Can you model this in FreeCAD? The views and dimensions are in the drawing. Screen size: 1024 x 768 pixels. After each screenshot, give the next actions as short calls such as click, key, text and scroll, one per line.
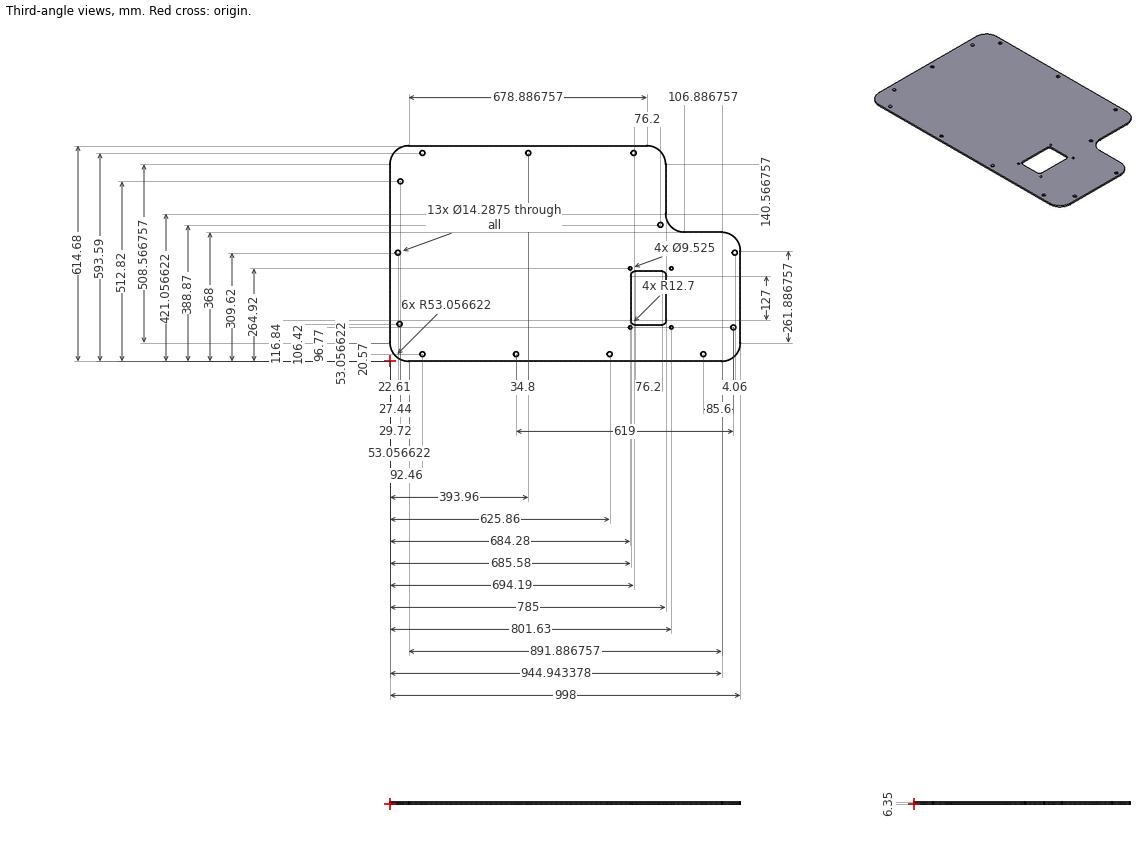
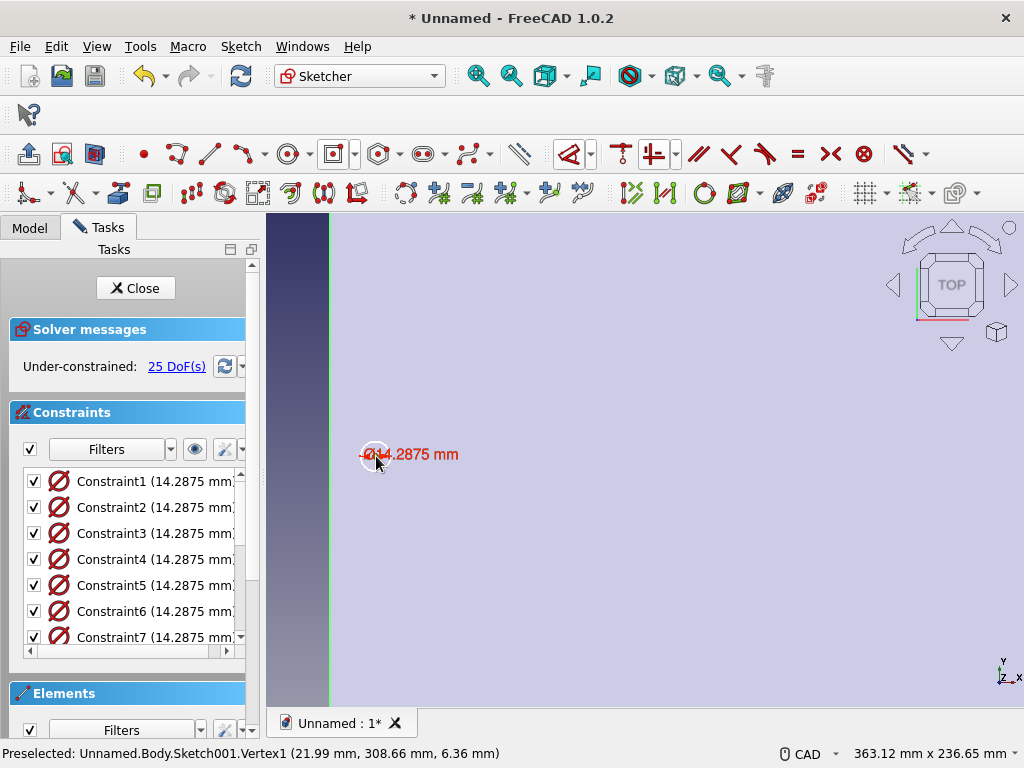
key(l)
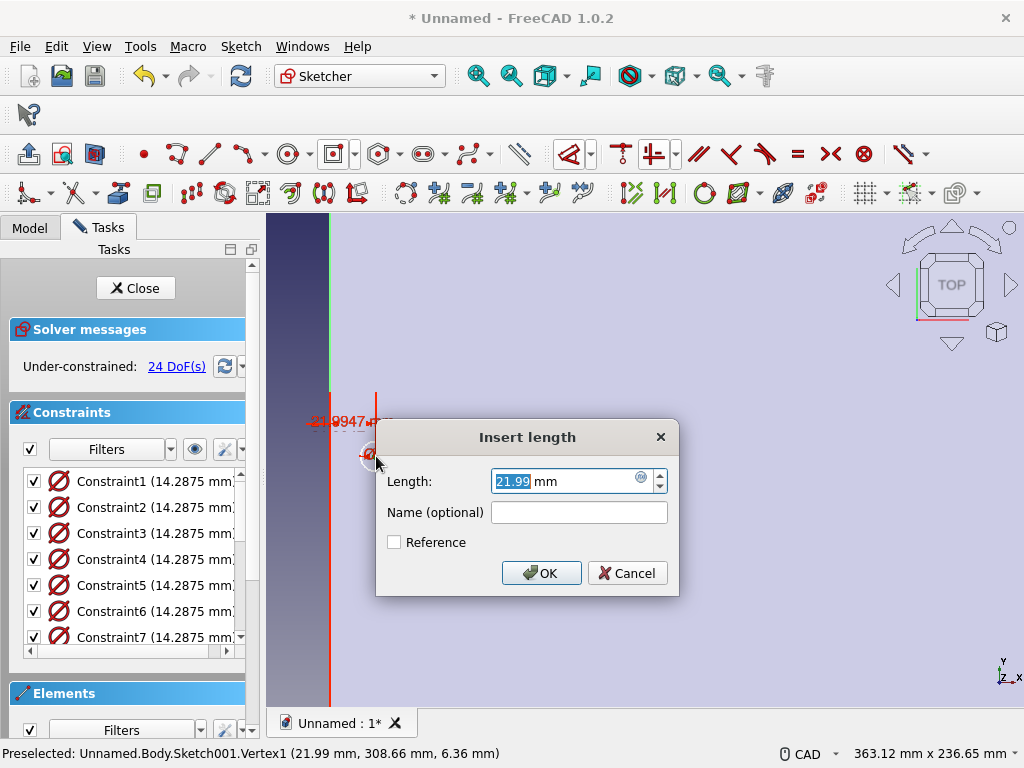
text(22.61)
key(Return)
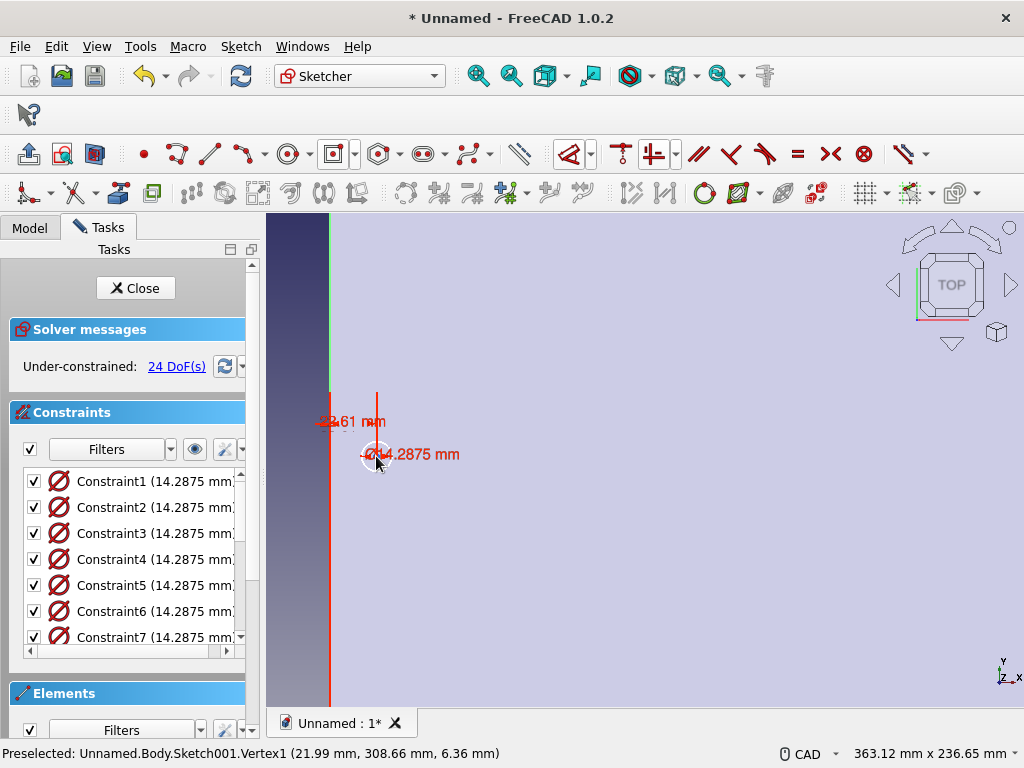
scroll(378, 457, down, 8)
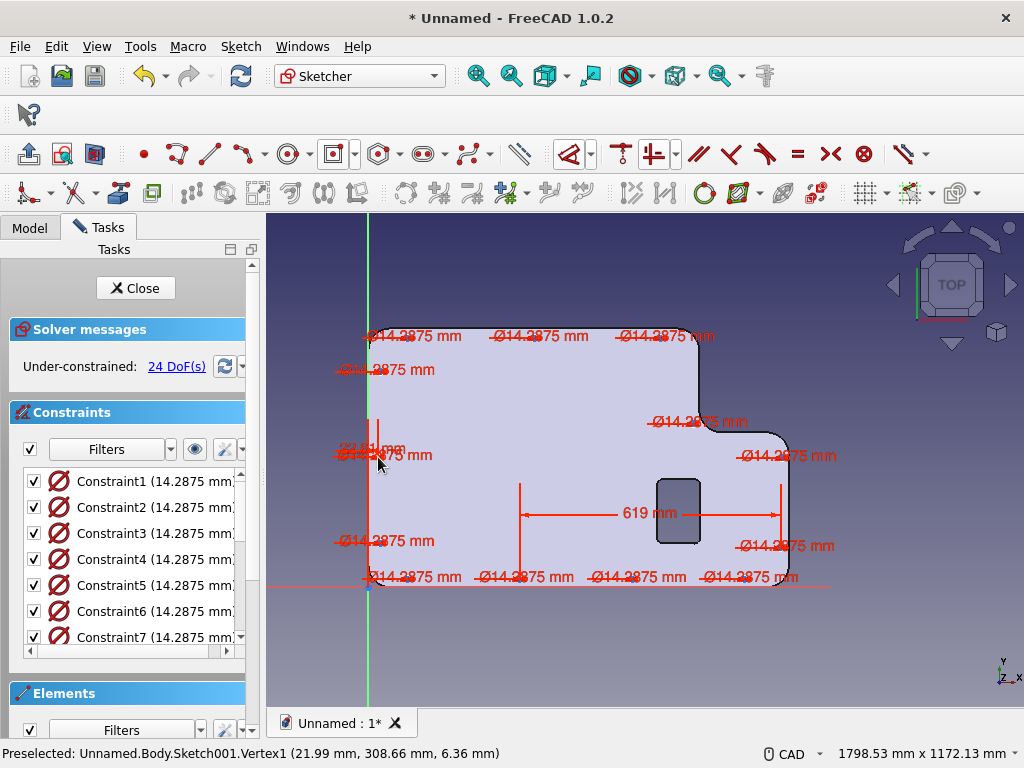
scroll(381, 372, up, 6)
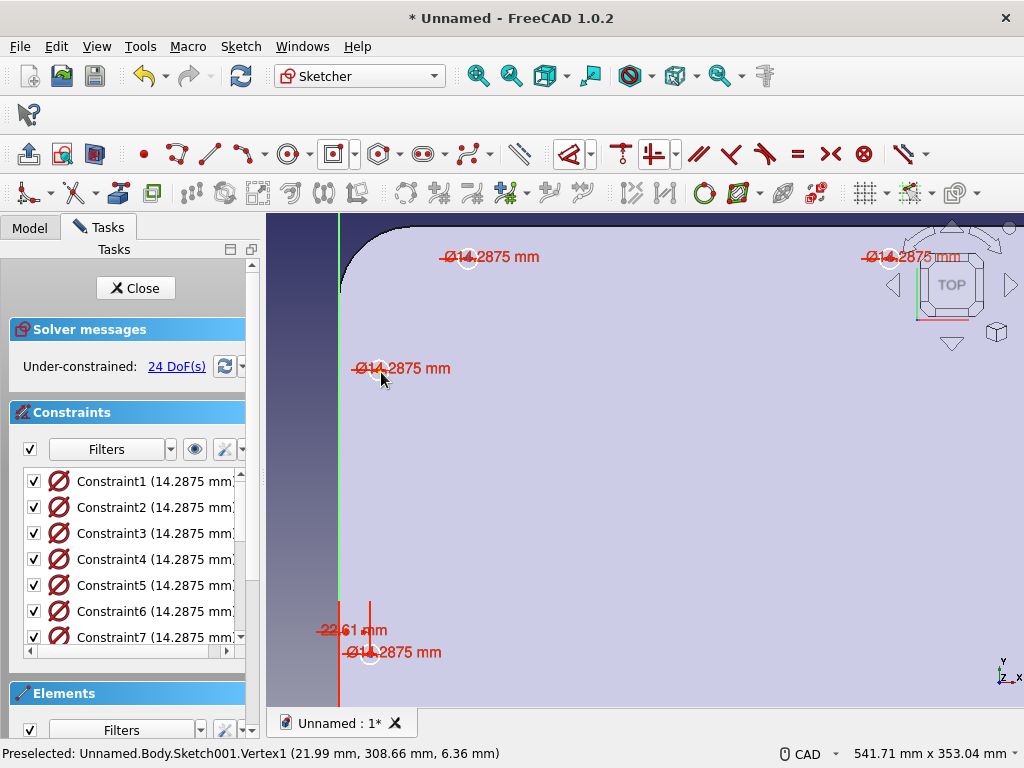
click(379, 370)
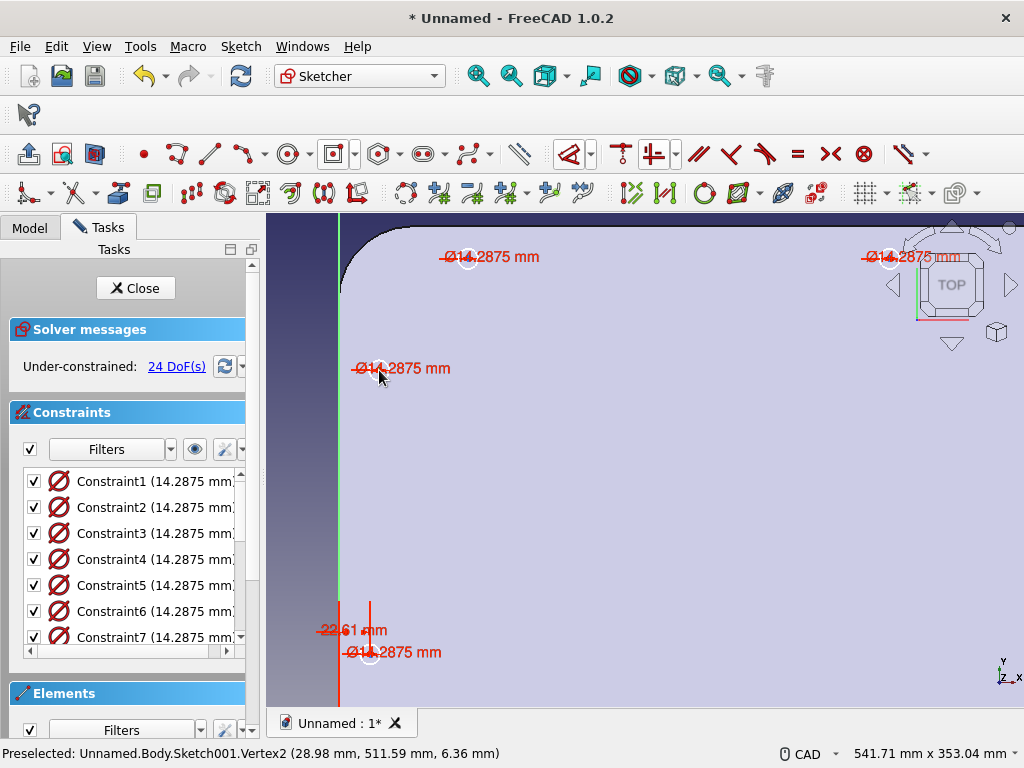
click(590, 154)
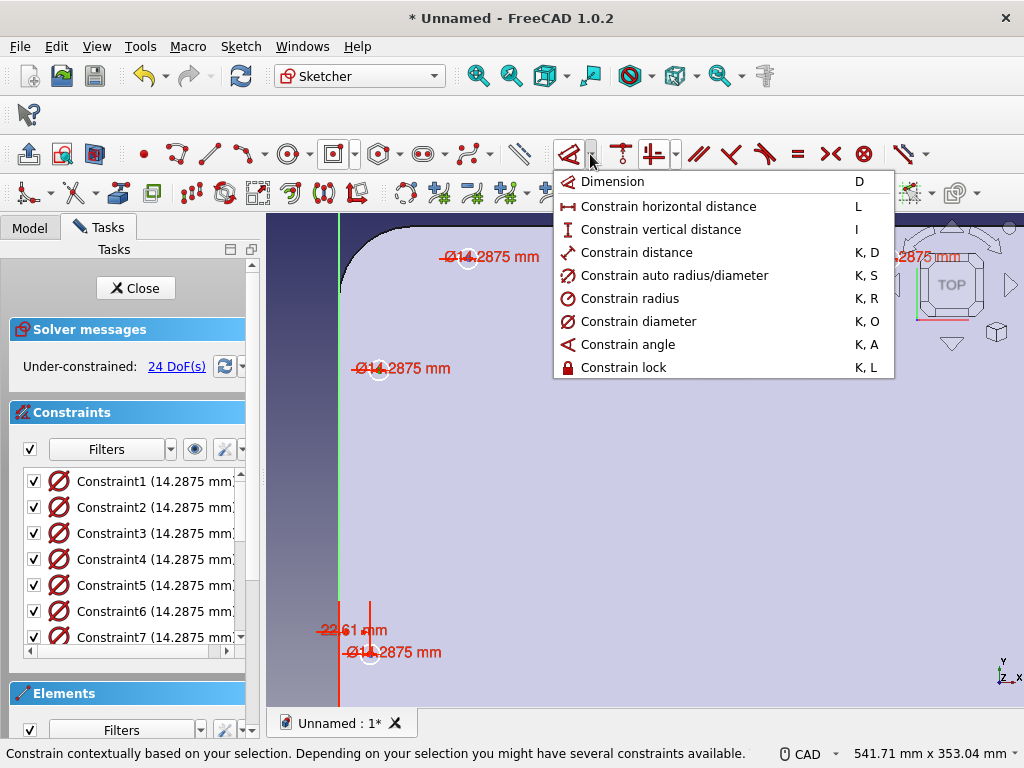
click(724, 206)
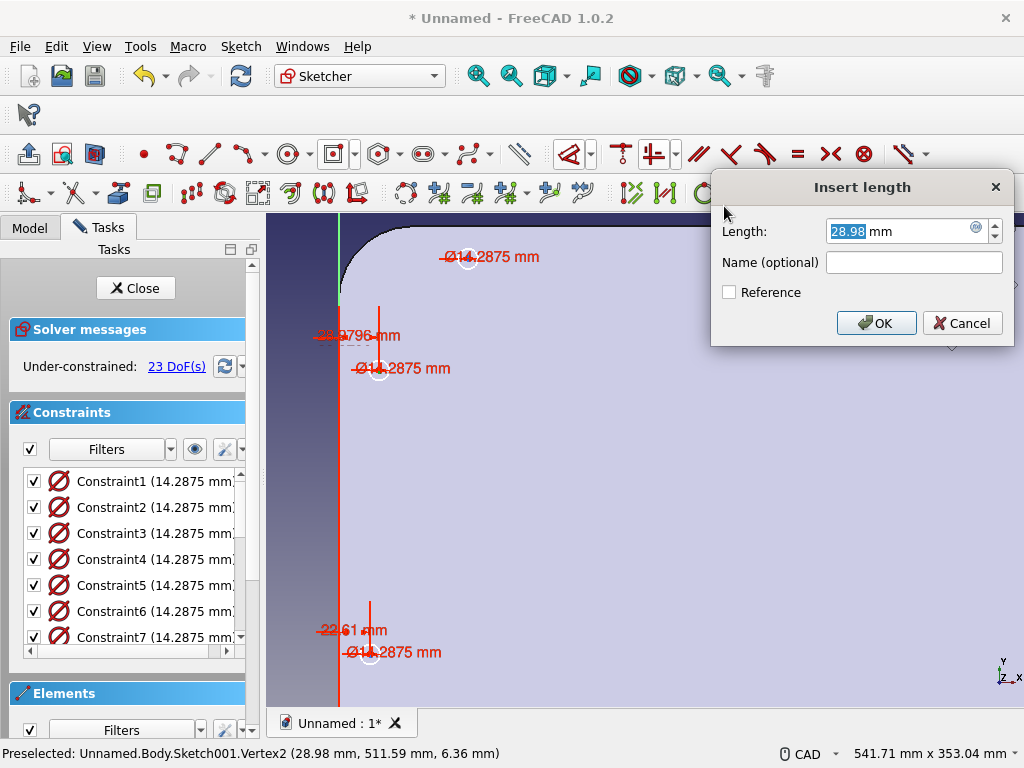
text(29.72)
key(Return)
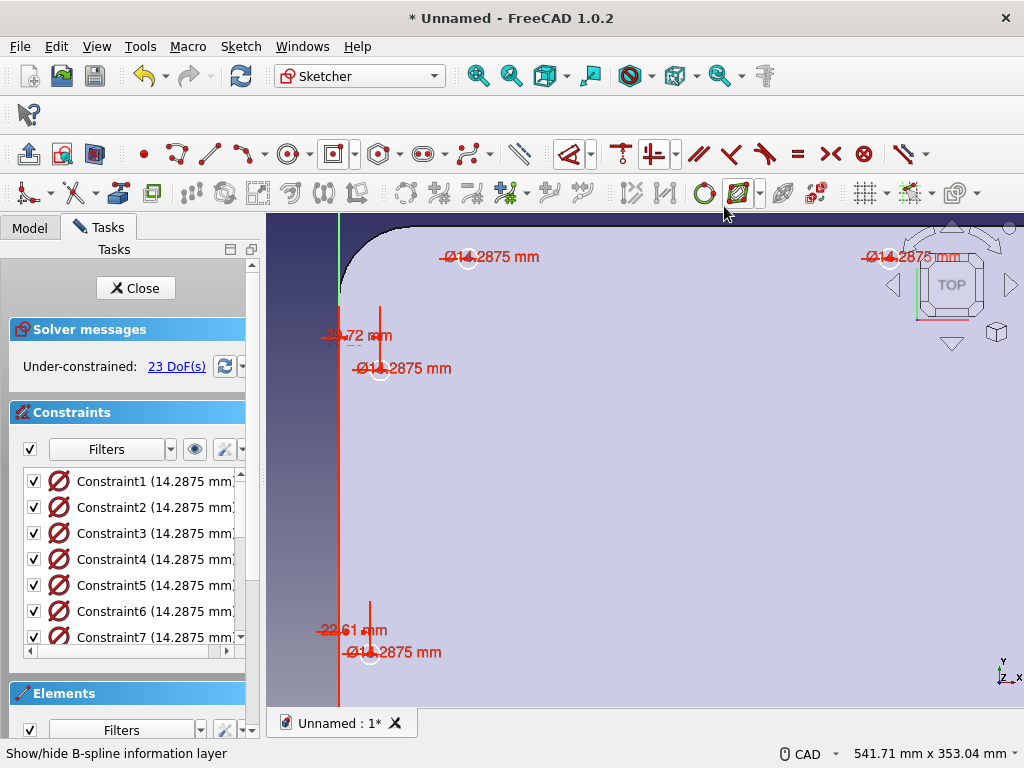
scroll(381, 371, down, 6)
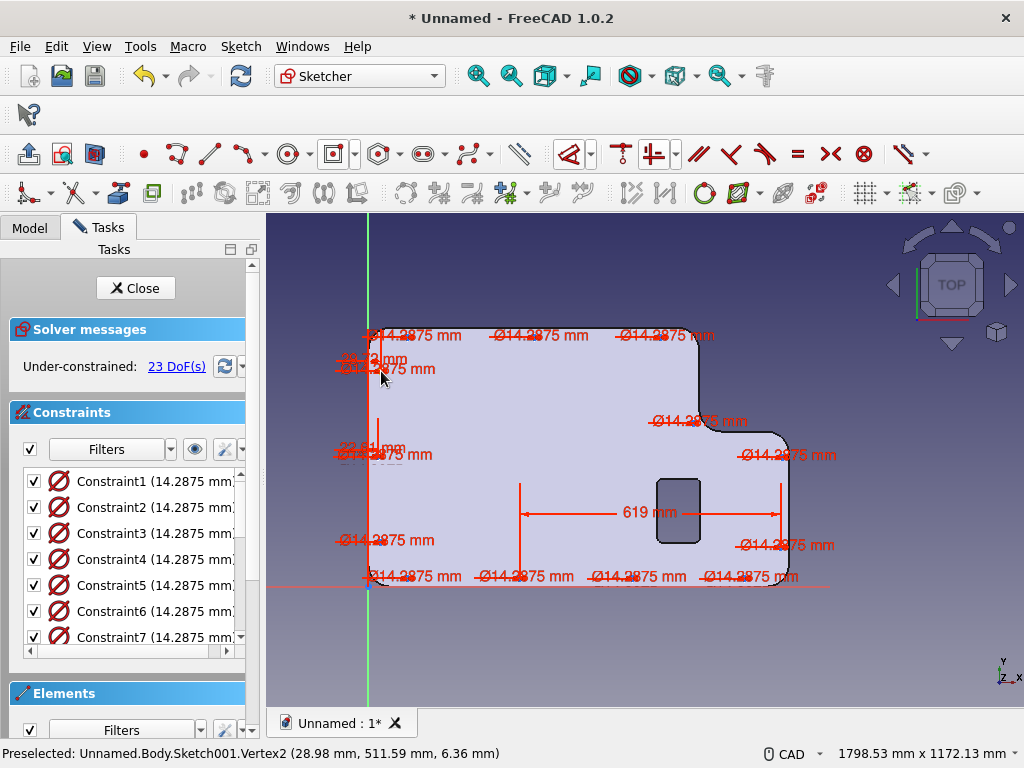
scroll(380, 542, up, 7)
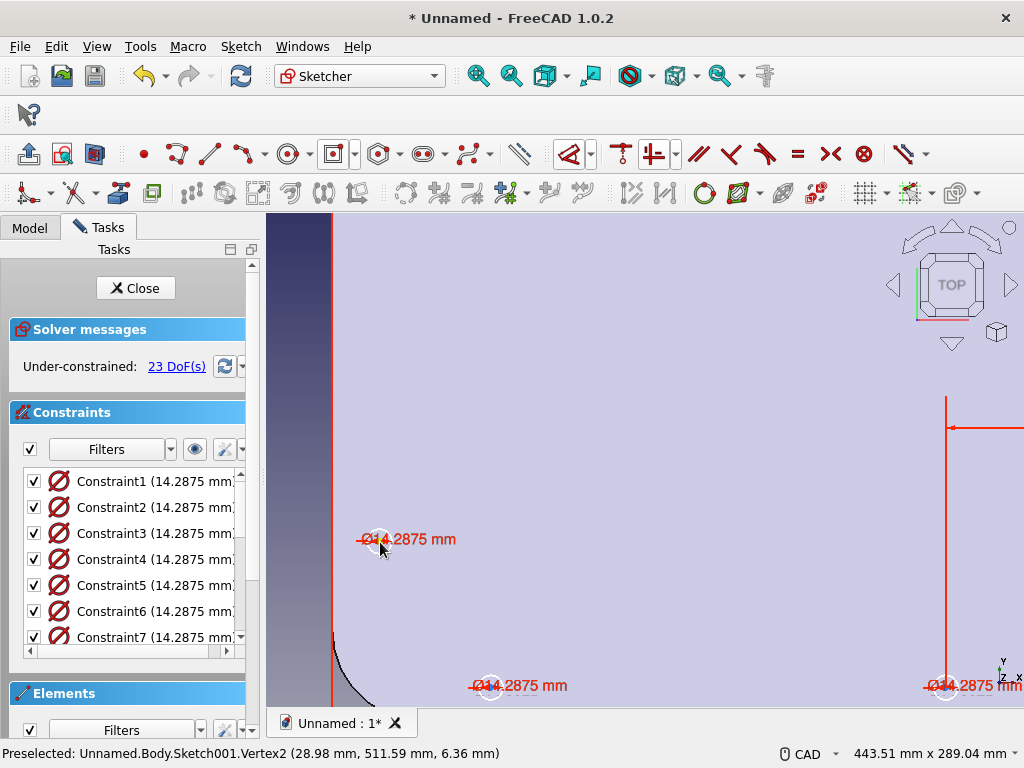
click(380, 541)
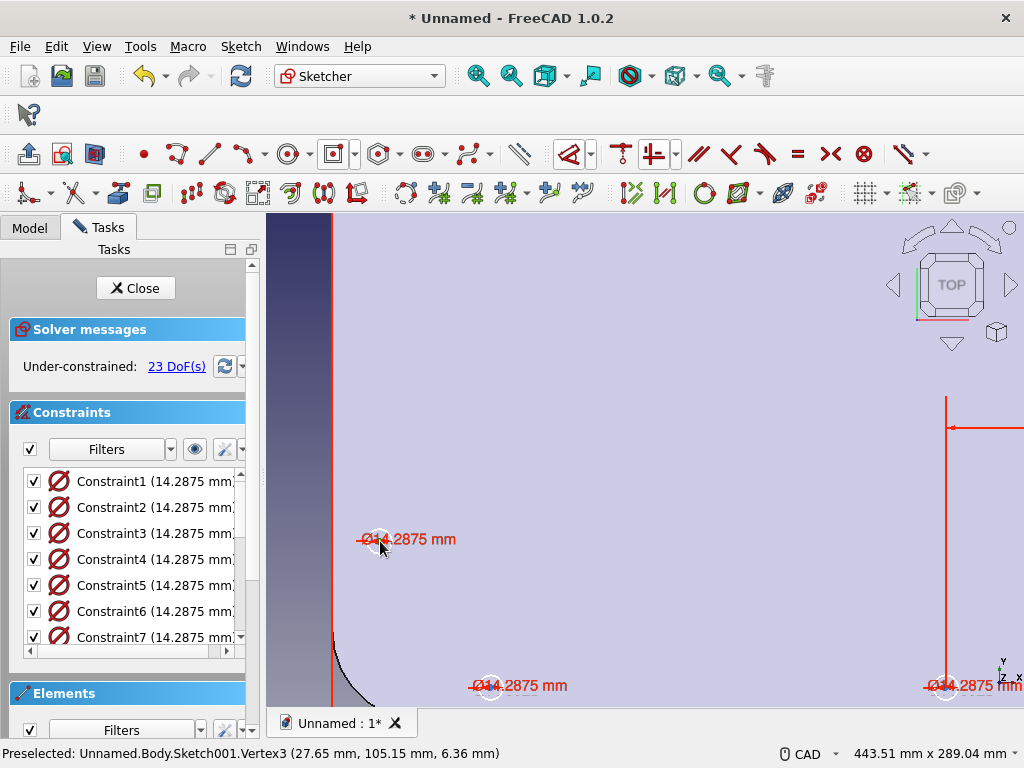
key(l)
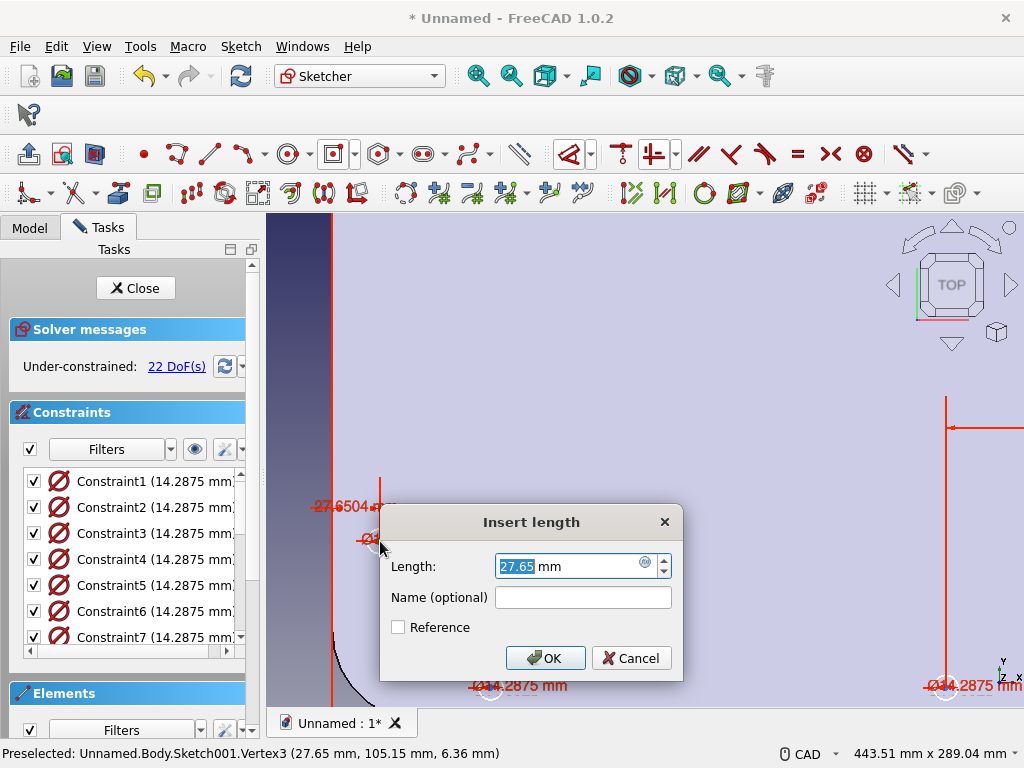
text(27.44)
key(Return)